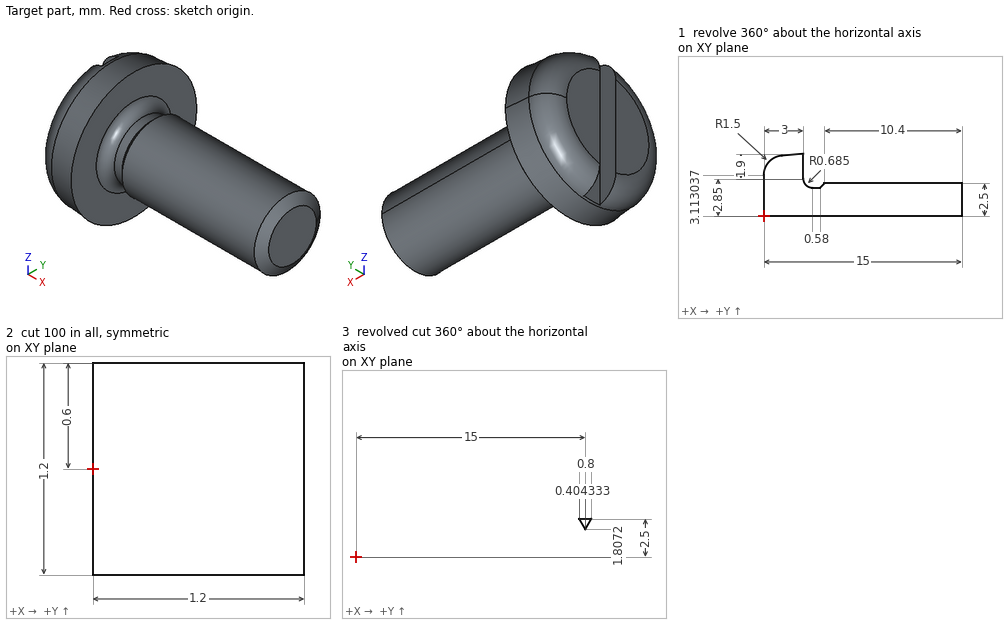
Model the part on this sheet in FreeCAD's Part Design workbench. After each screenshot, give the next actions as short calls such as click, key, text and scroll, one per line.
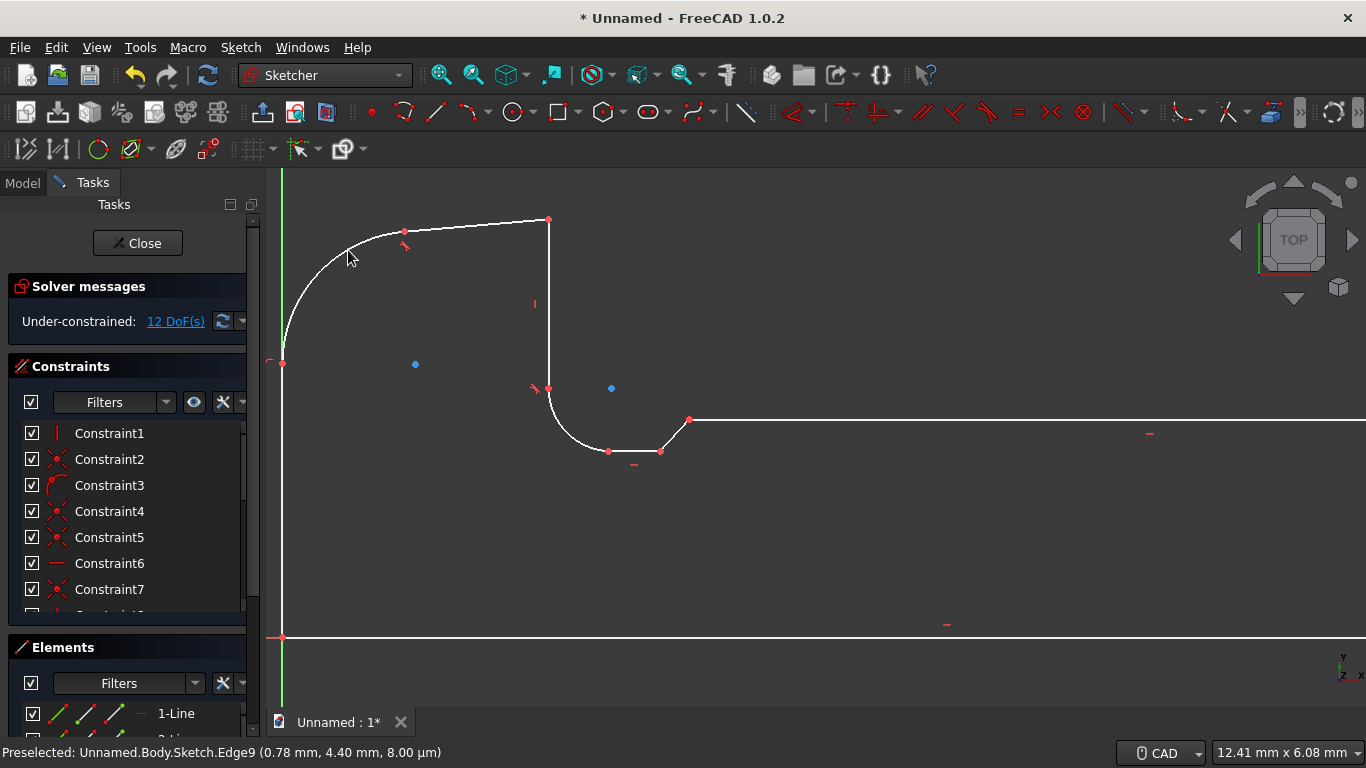
scroll(585, 446, down, 4)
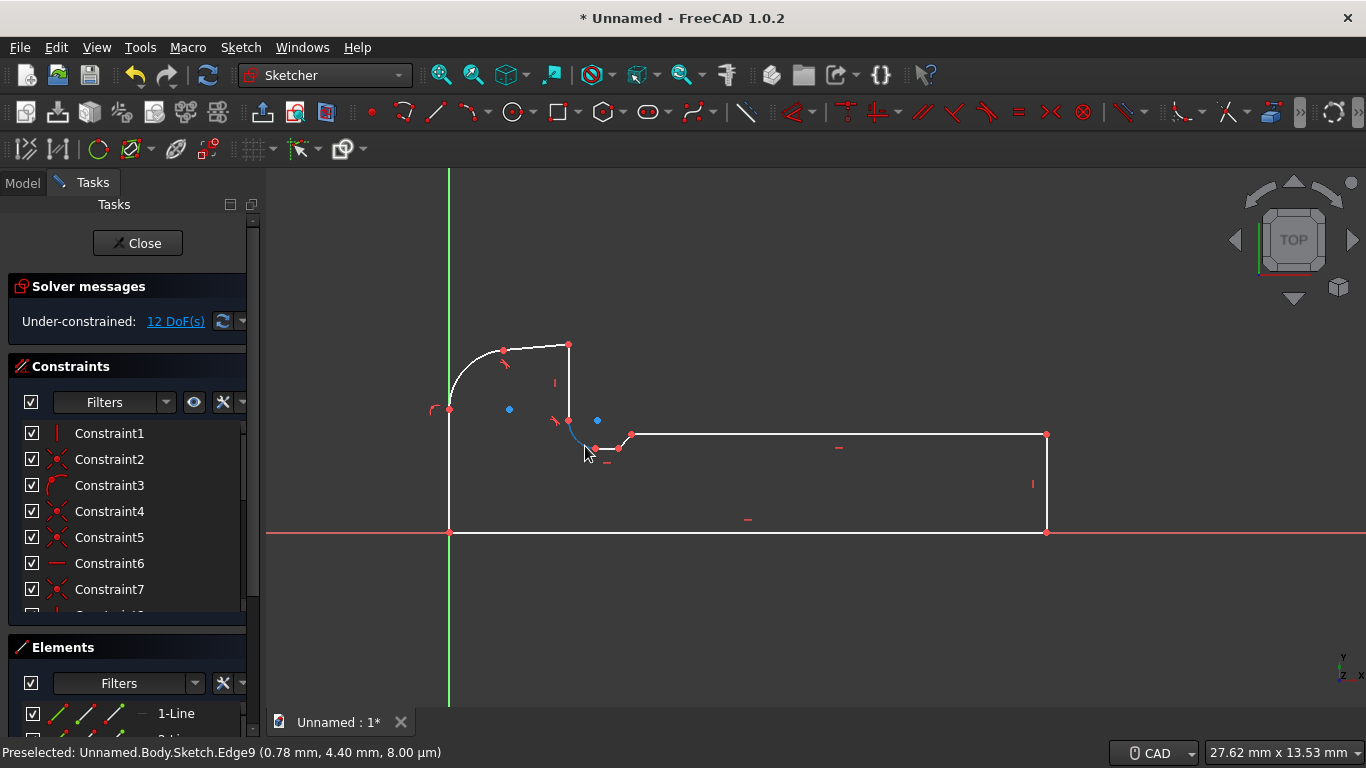
click(449, 446)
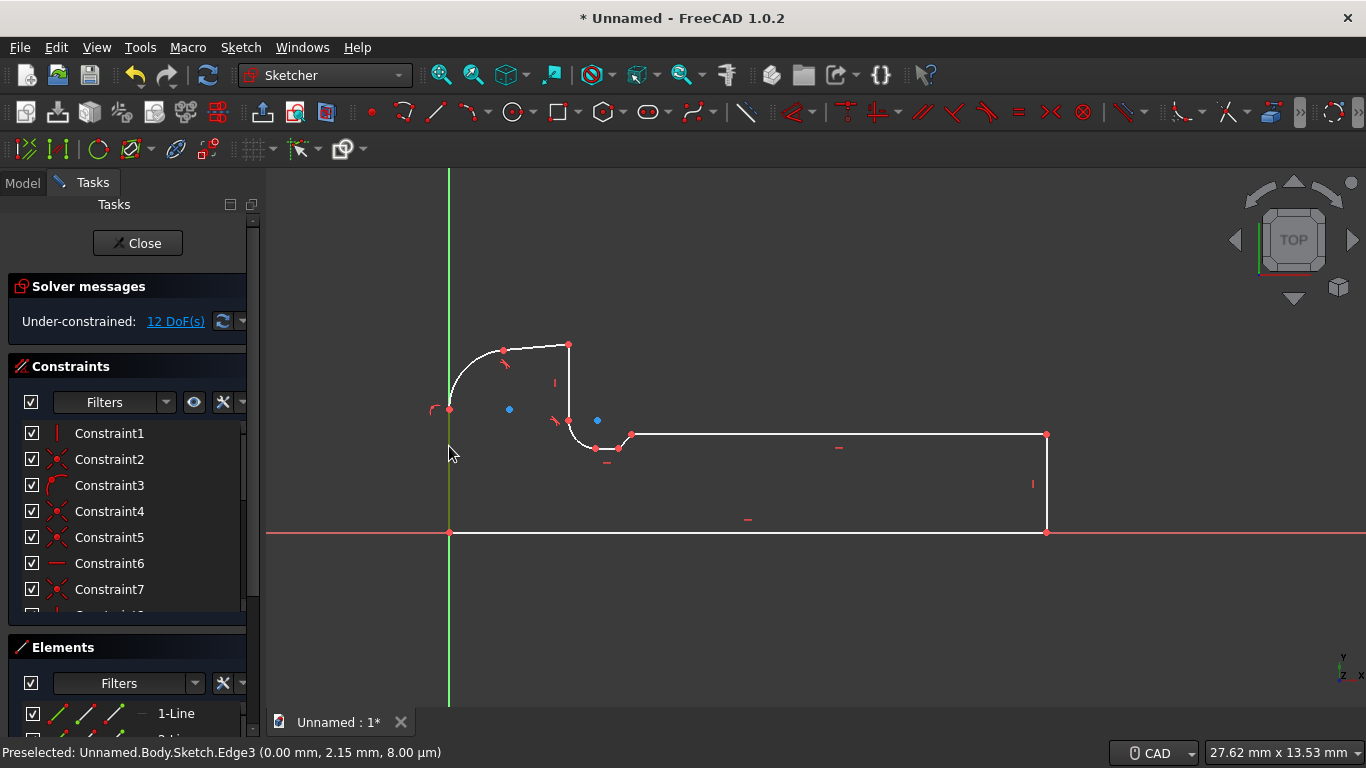
click(479, 358)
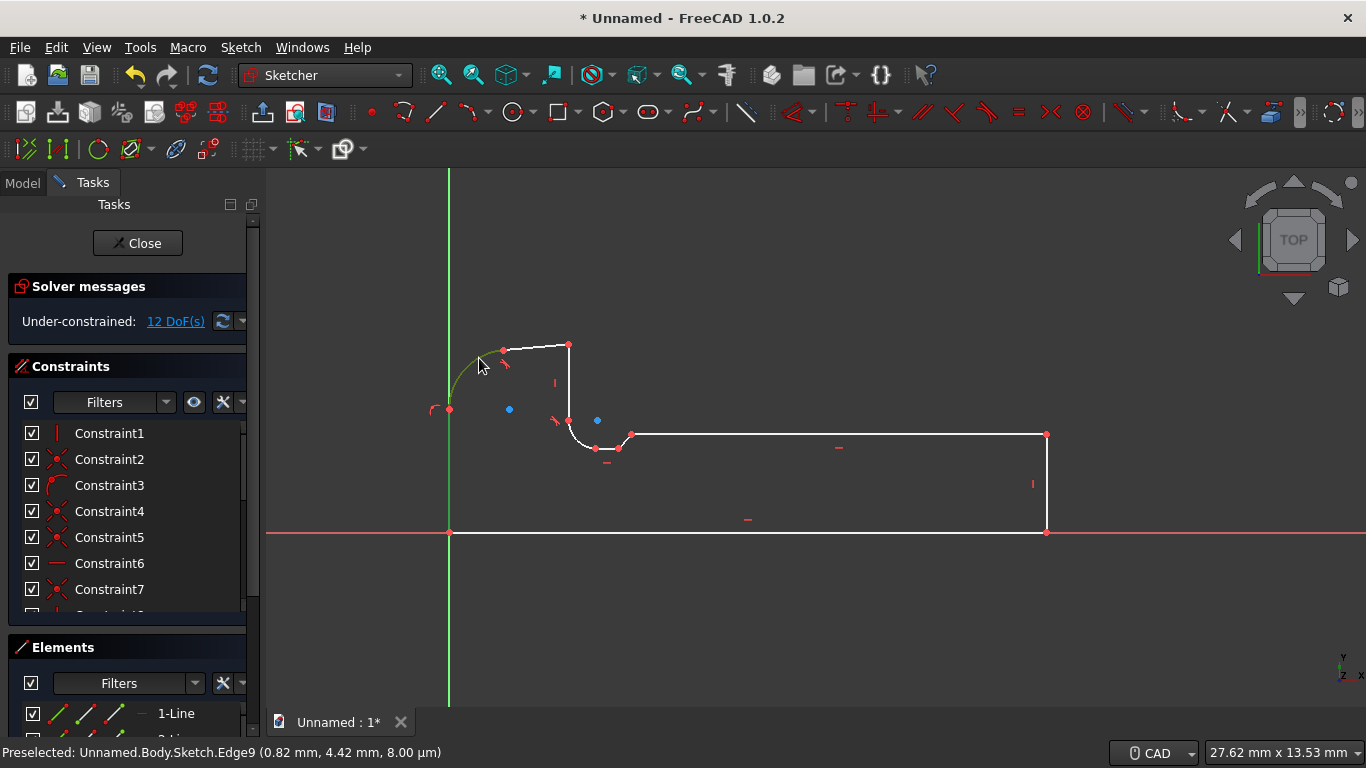
key(t)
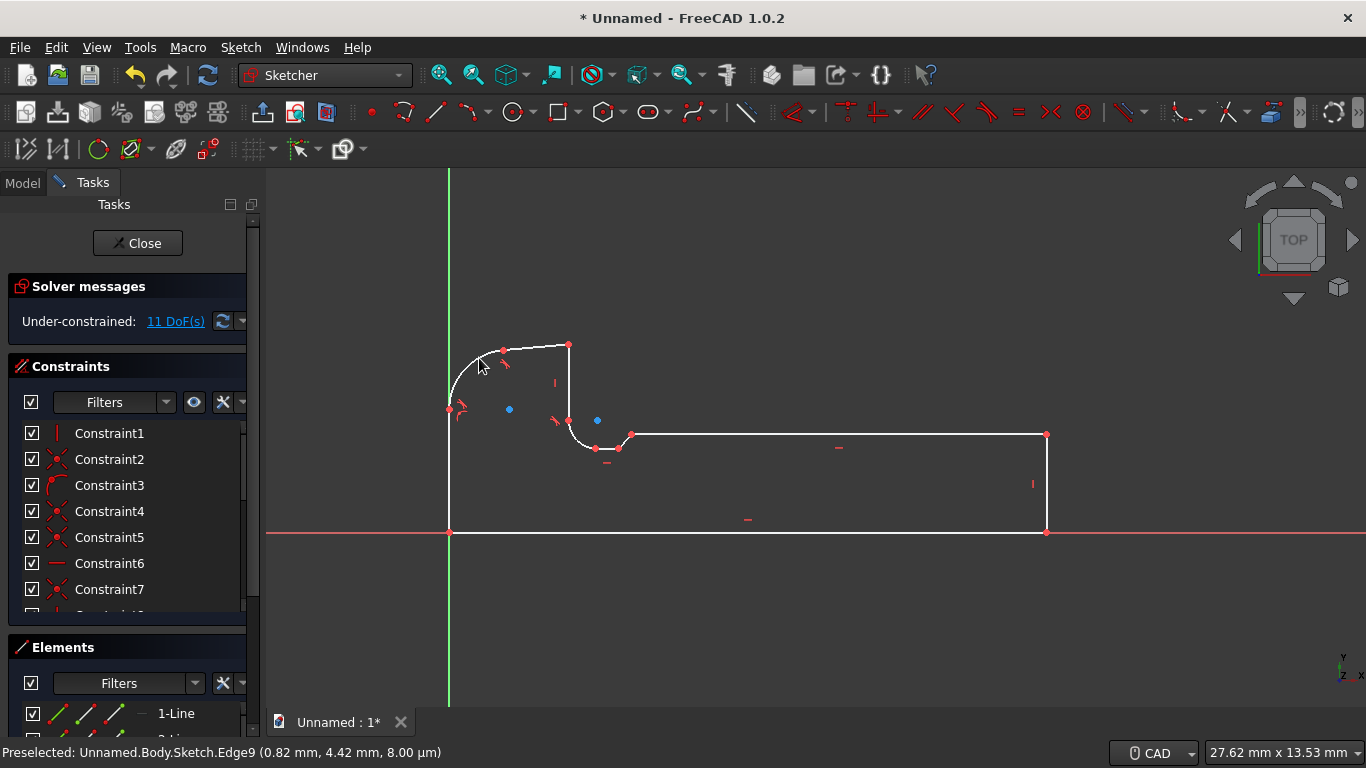
scroll(610, 449, up, 3)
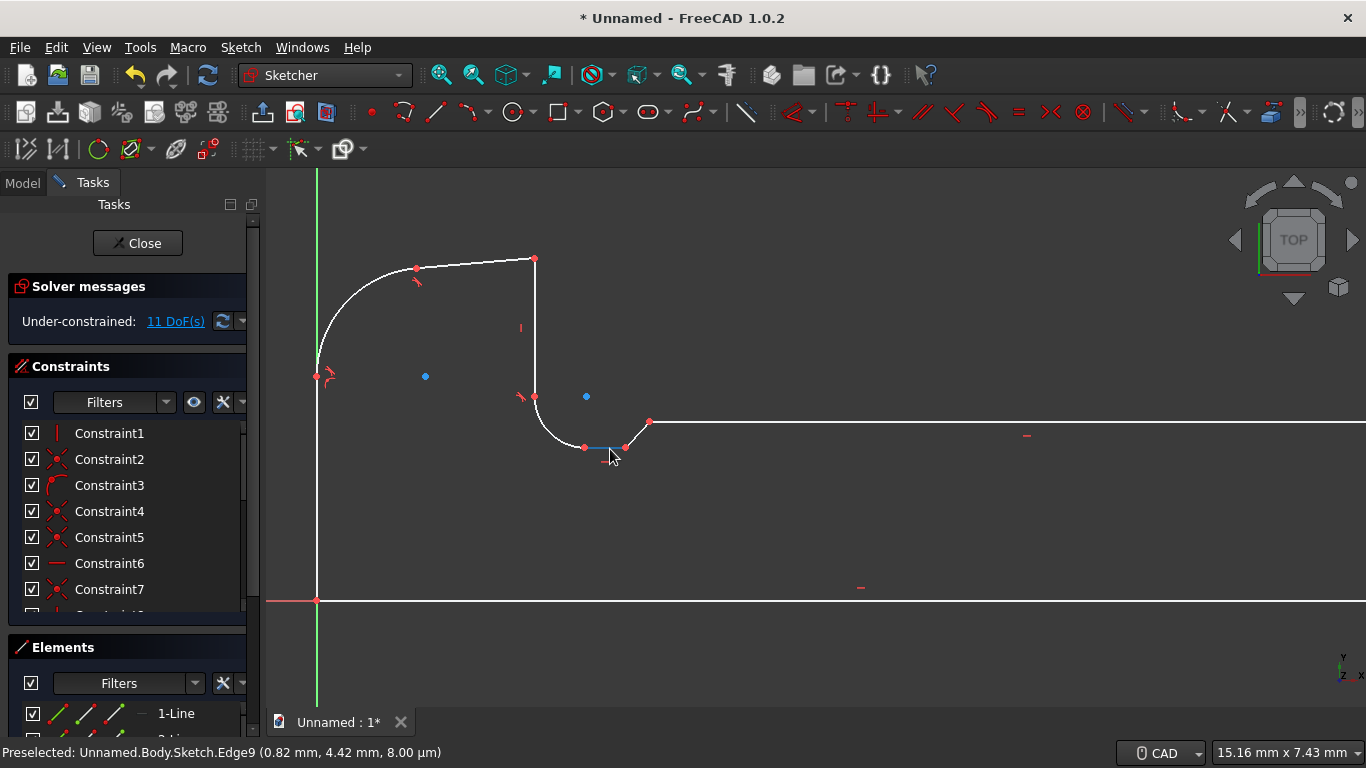
click(609, 448)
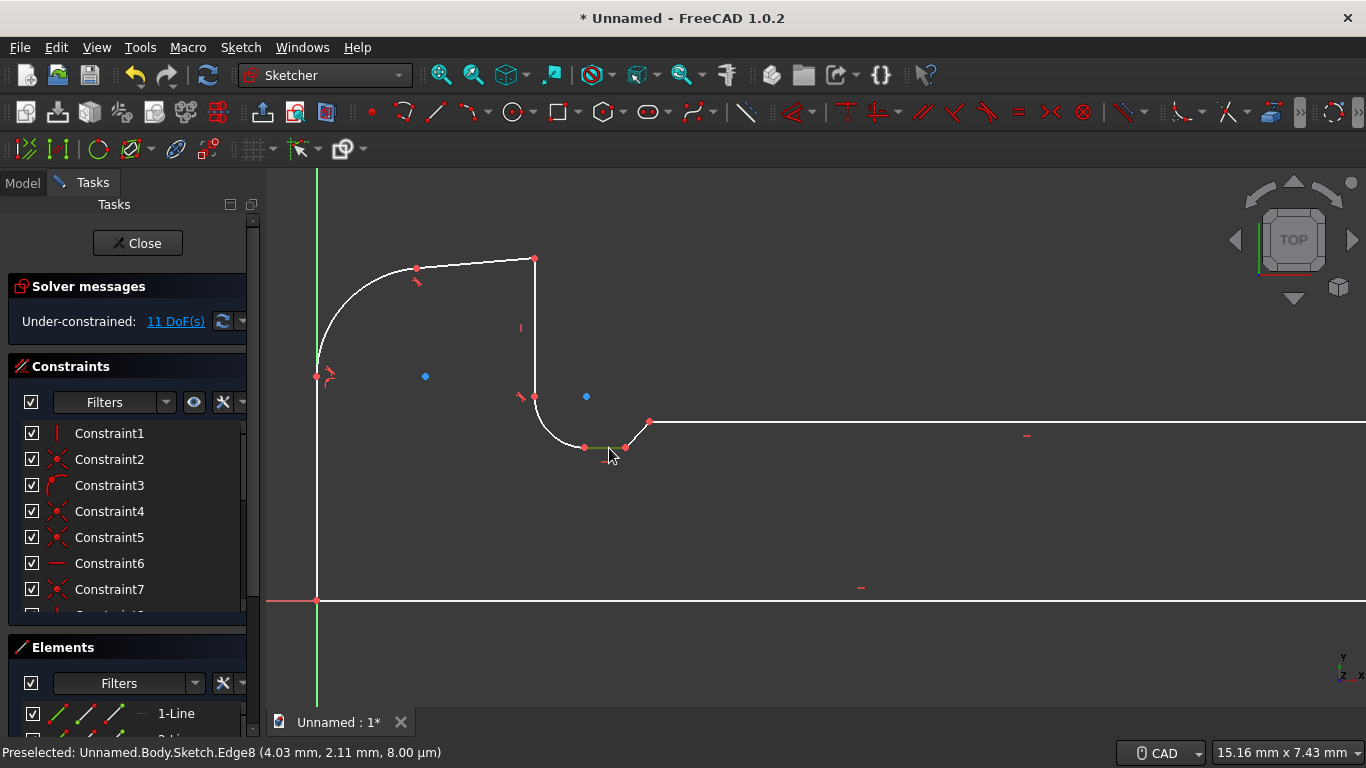
click(540, 419)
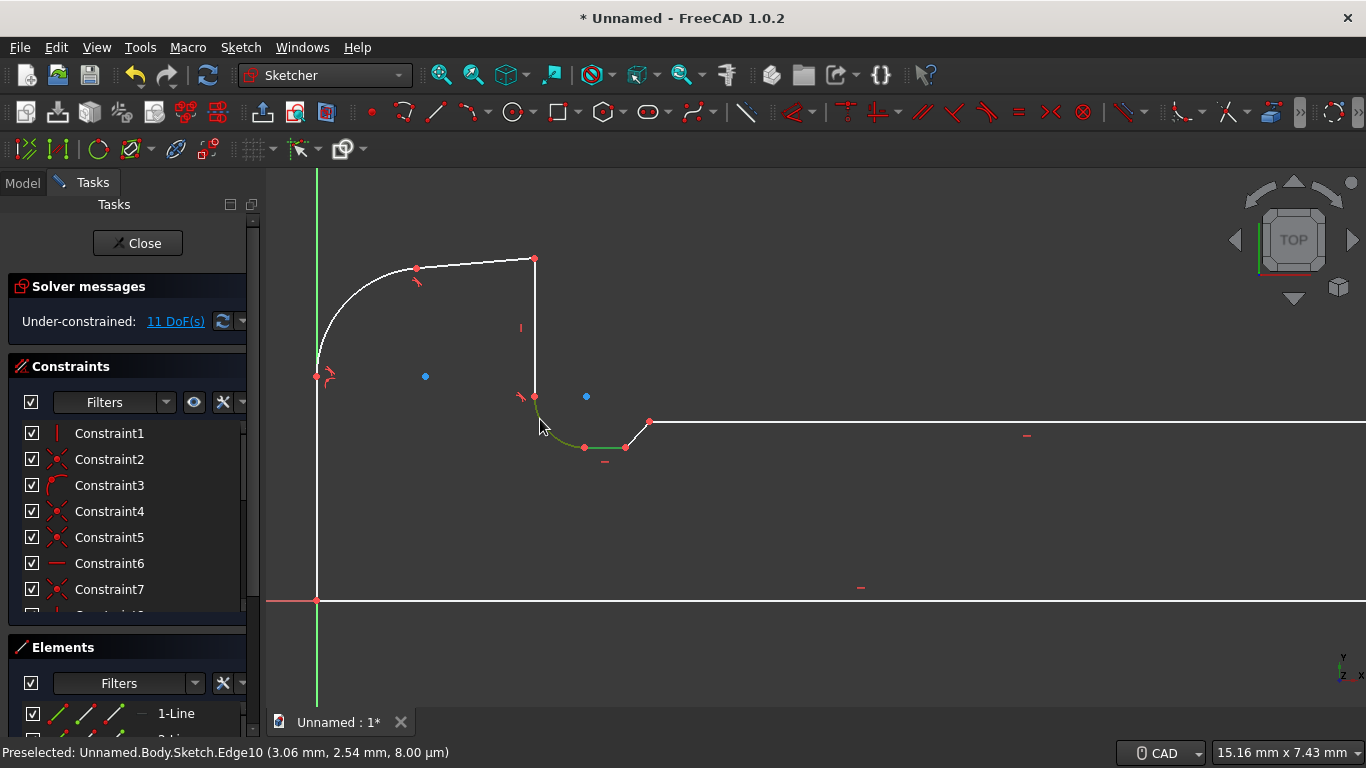
key(t)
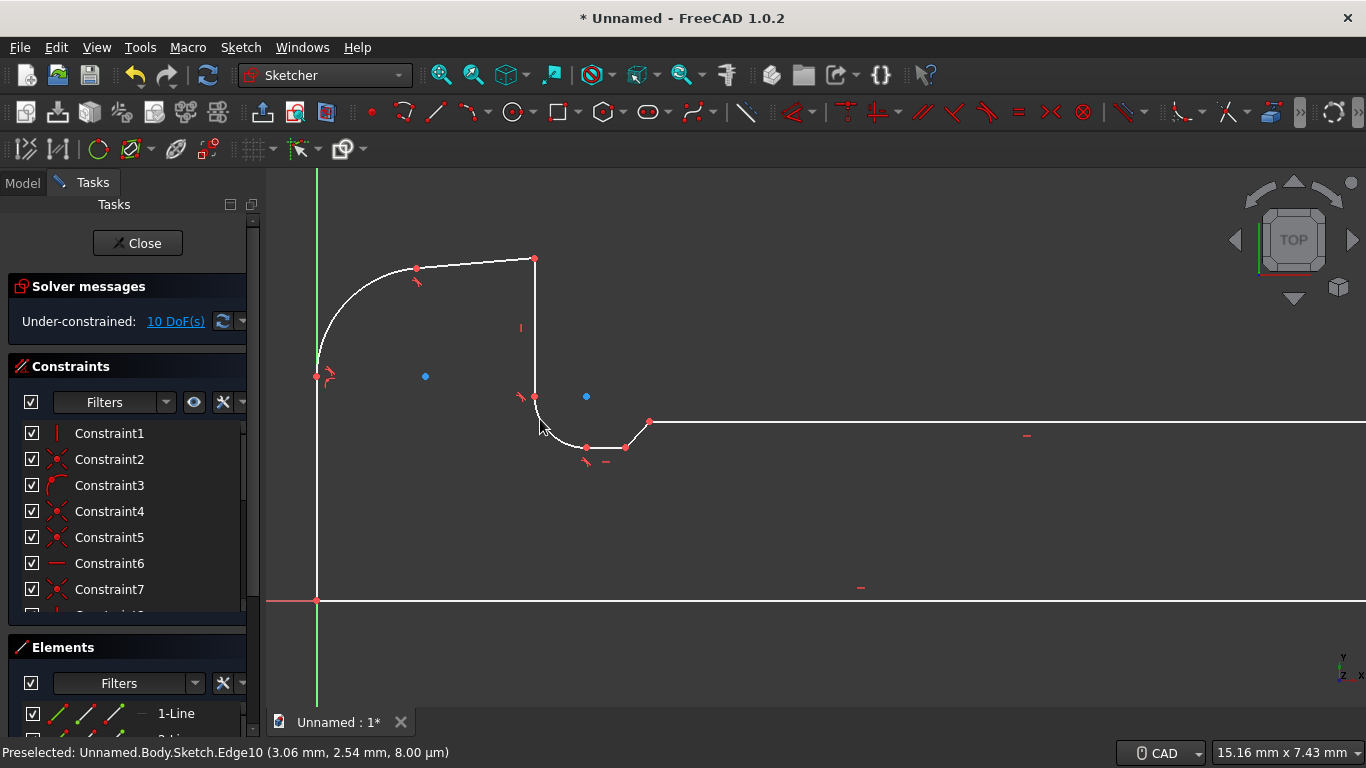
key(d)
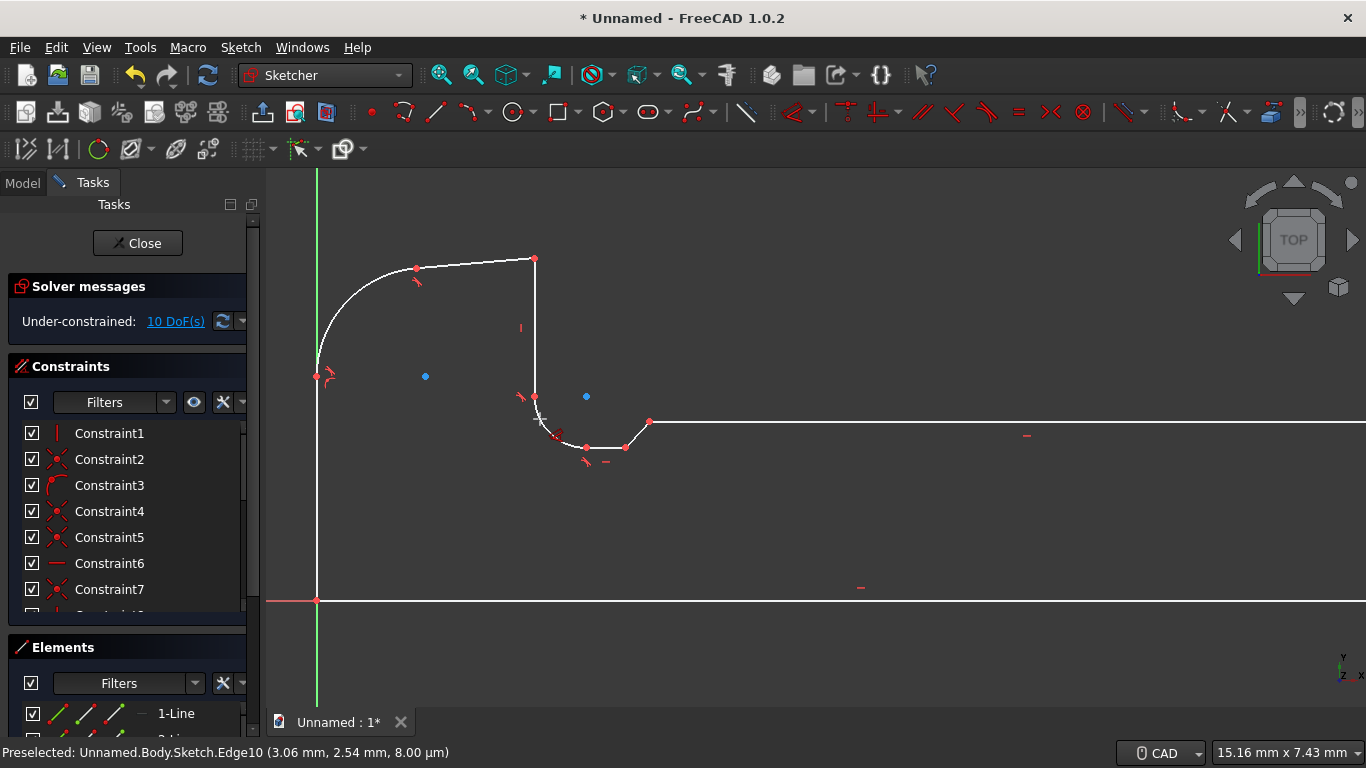
click(371, 283)
click(355, 255)